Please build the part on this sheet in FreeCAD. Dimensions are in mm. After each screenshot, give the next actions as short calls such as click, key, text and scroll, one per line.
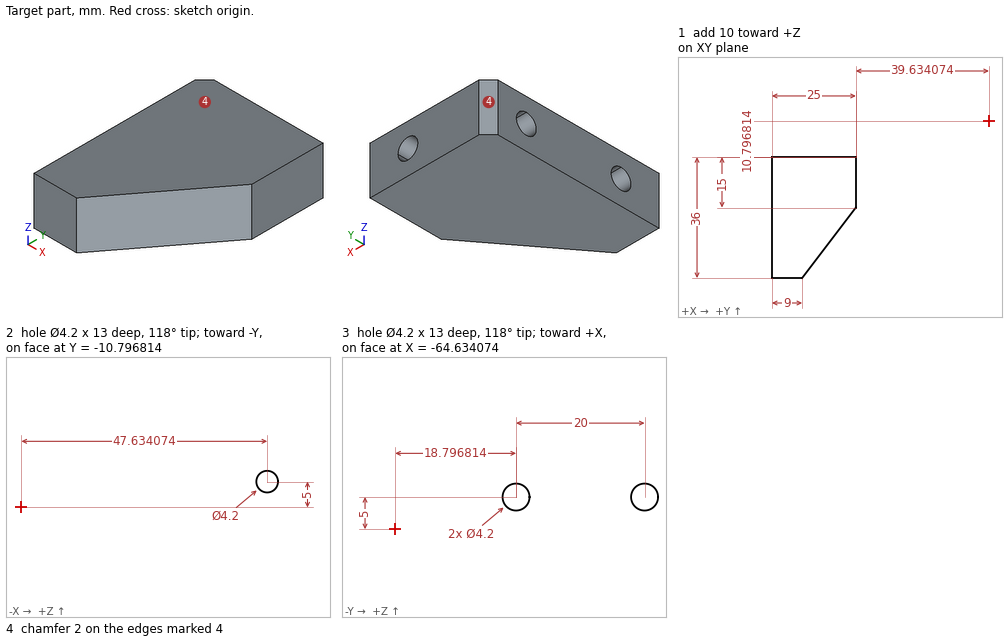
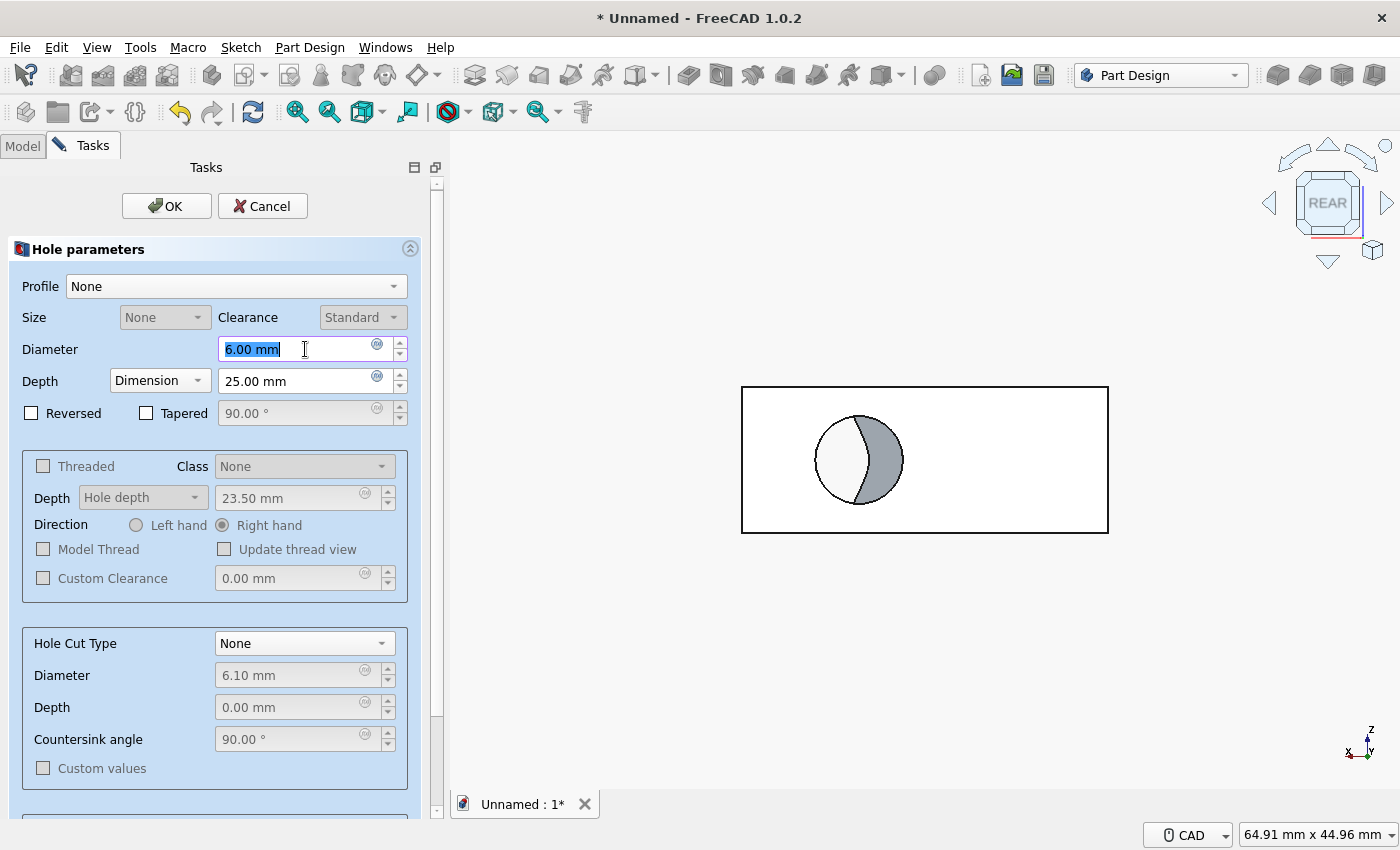
text(4.2)
key(Tab)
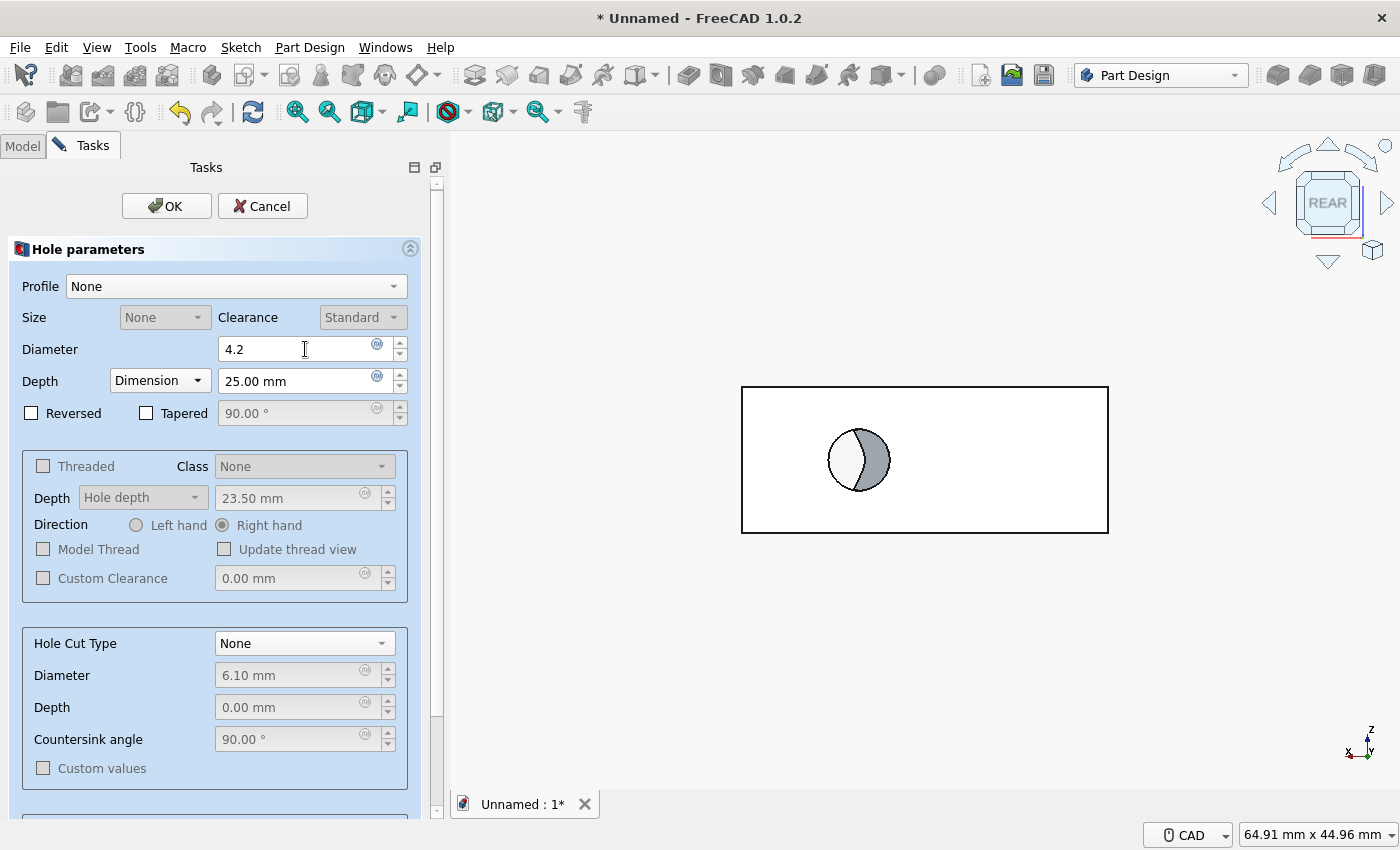
triple_click(305, 381)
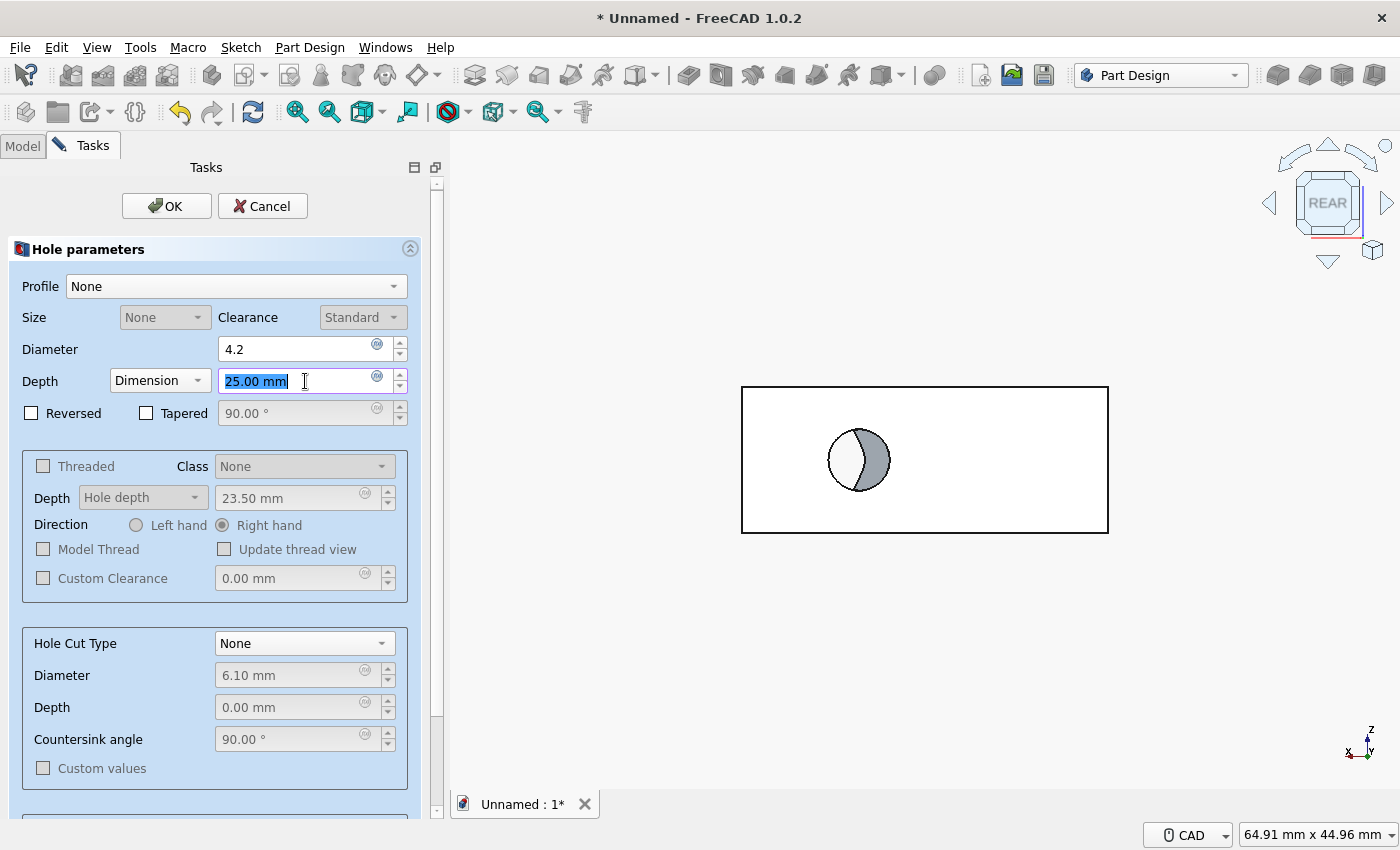
text(13)
key(Tab)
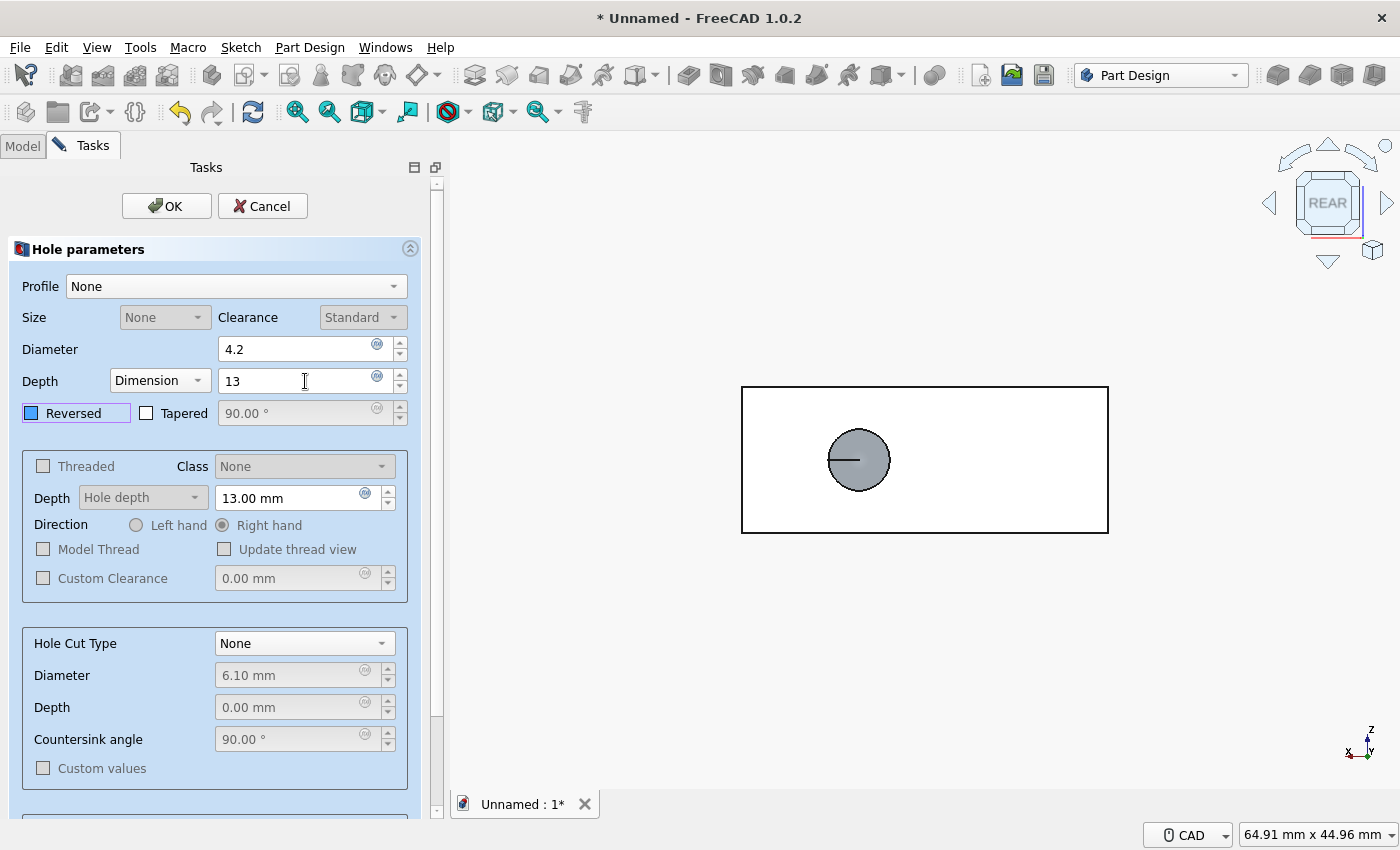
click(167, 206)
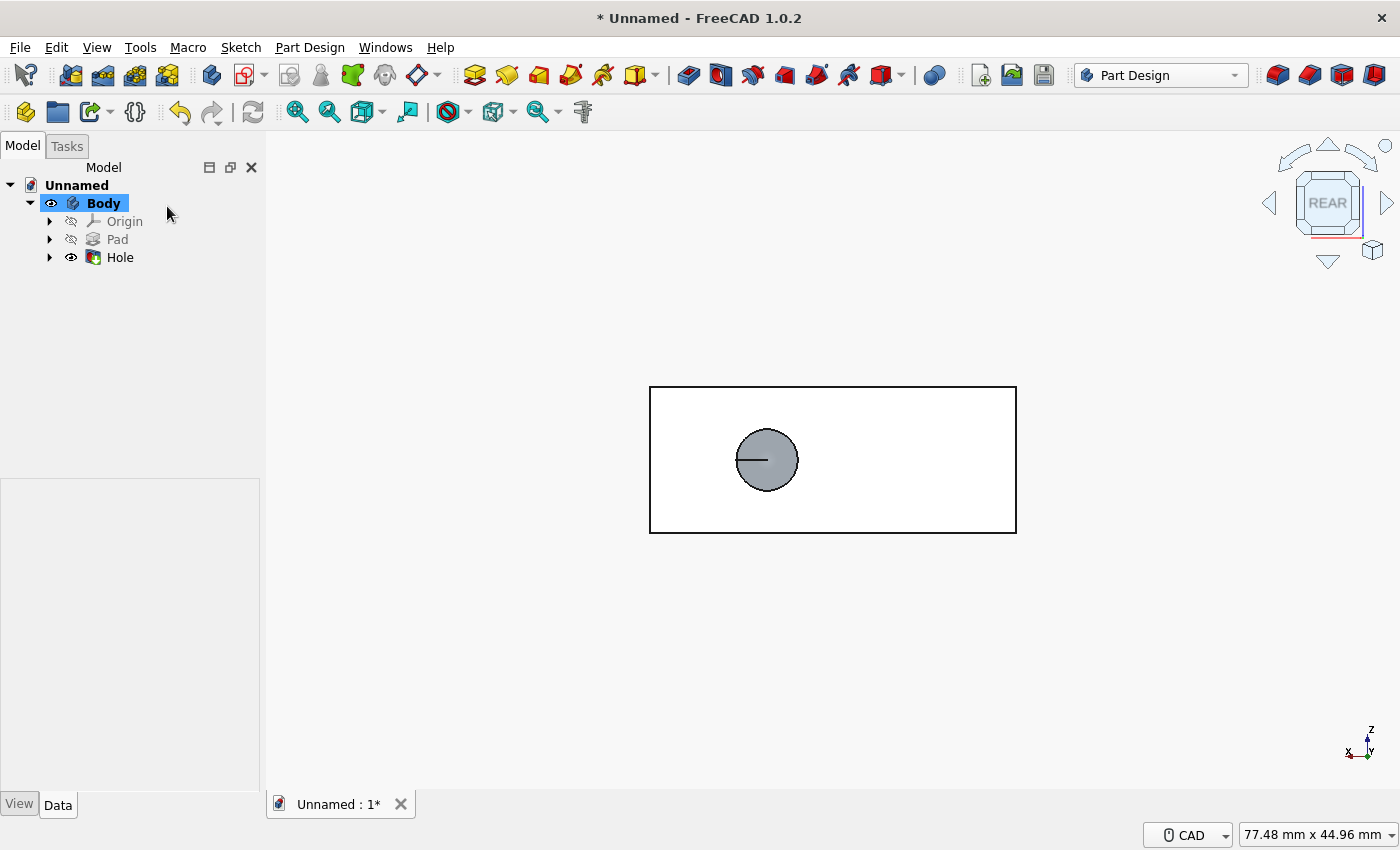
click(298, 112)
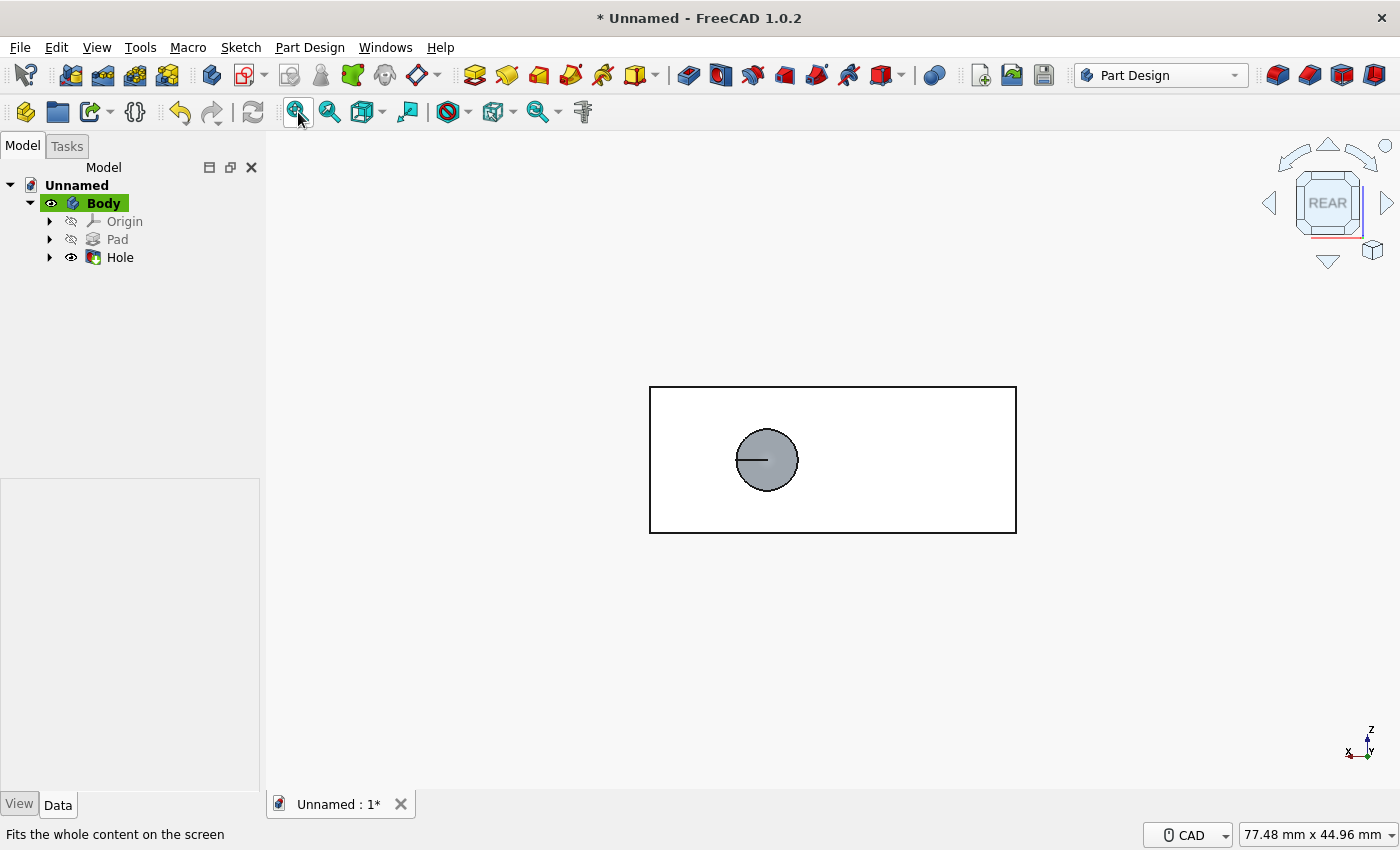
key(6)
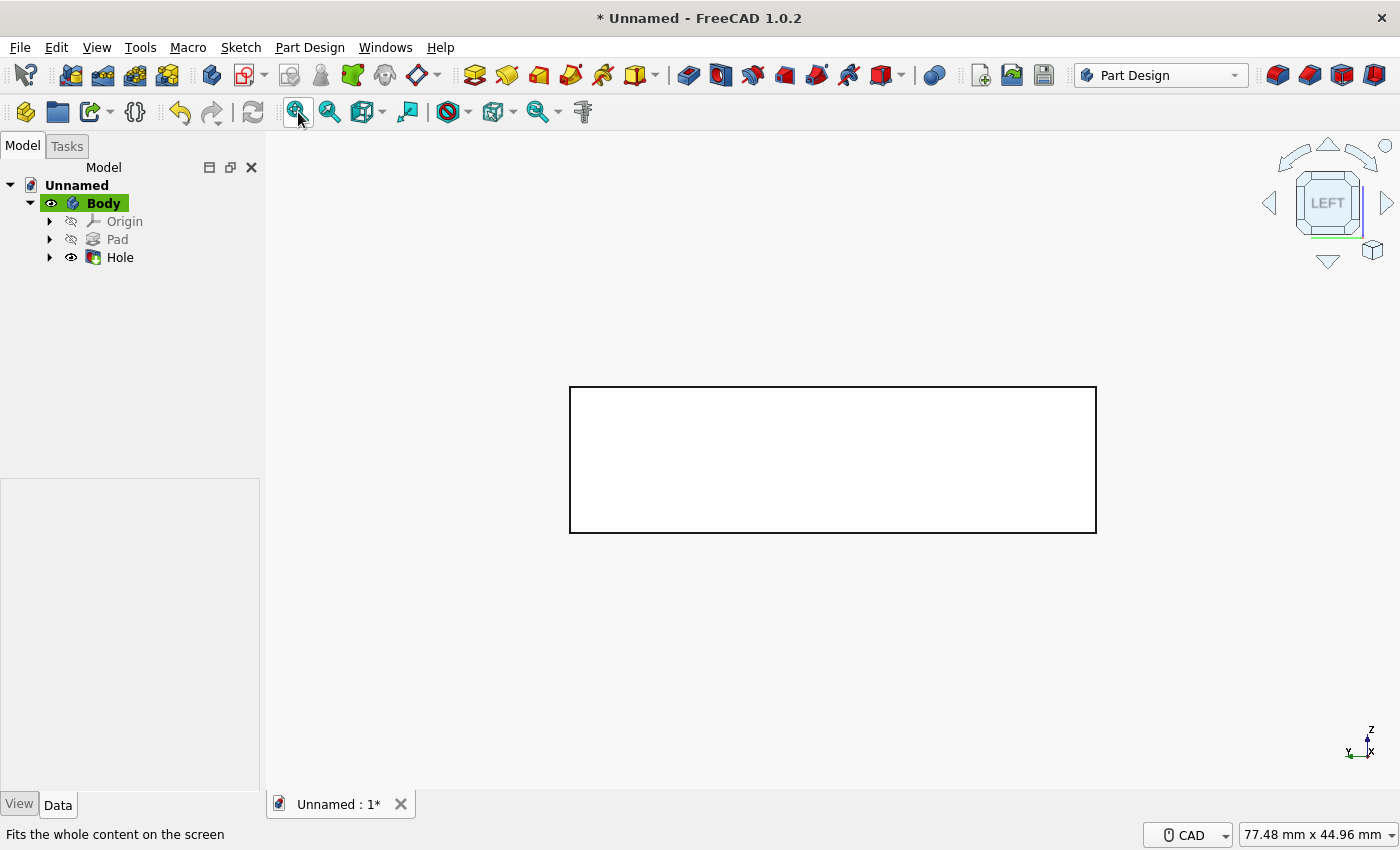
click(682, 459)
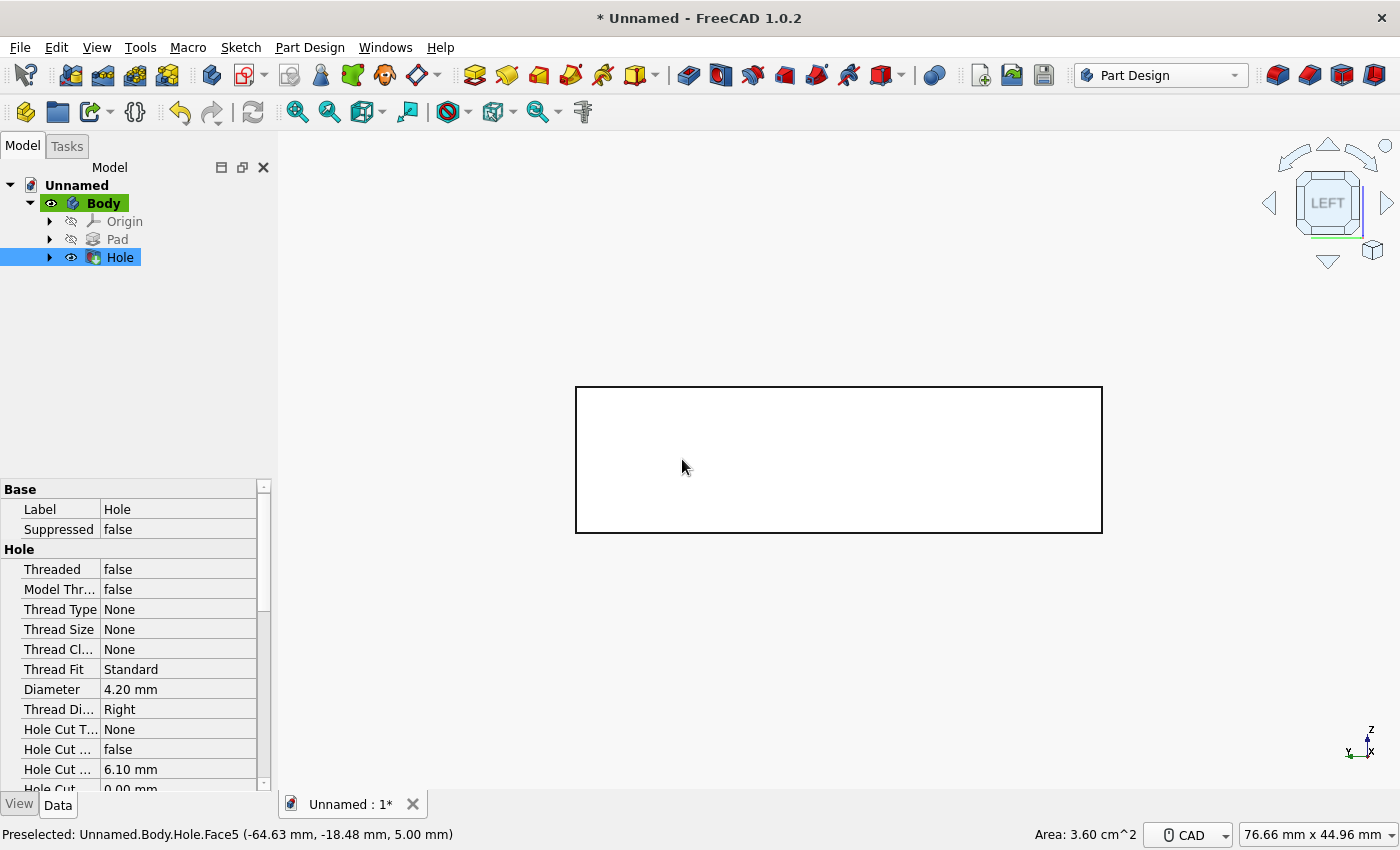
click(244, 76)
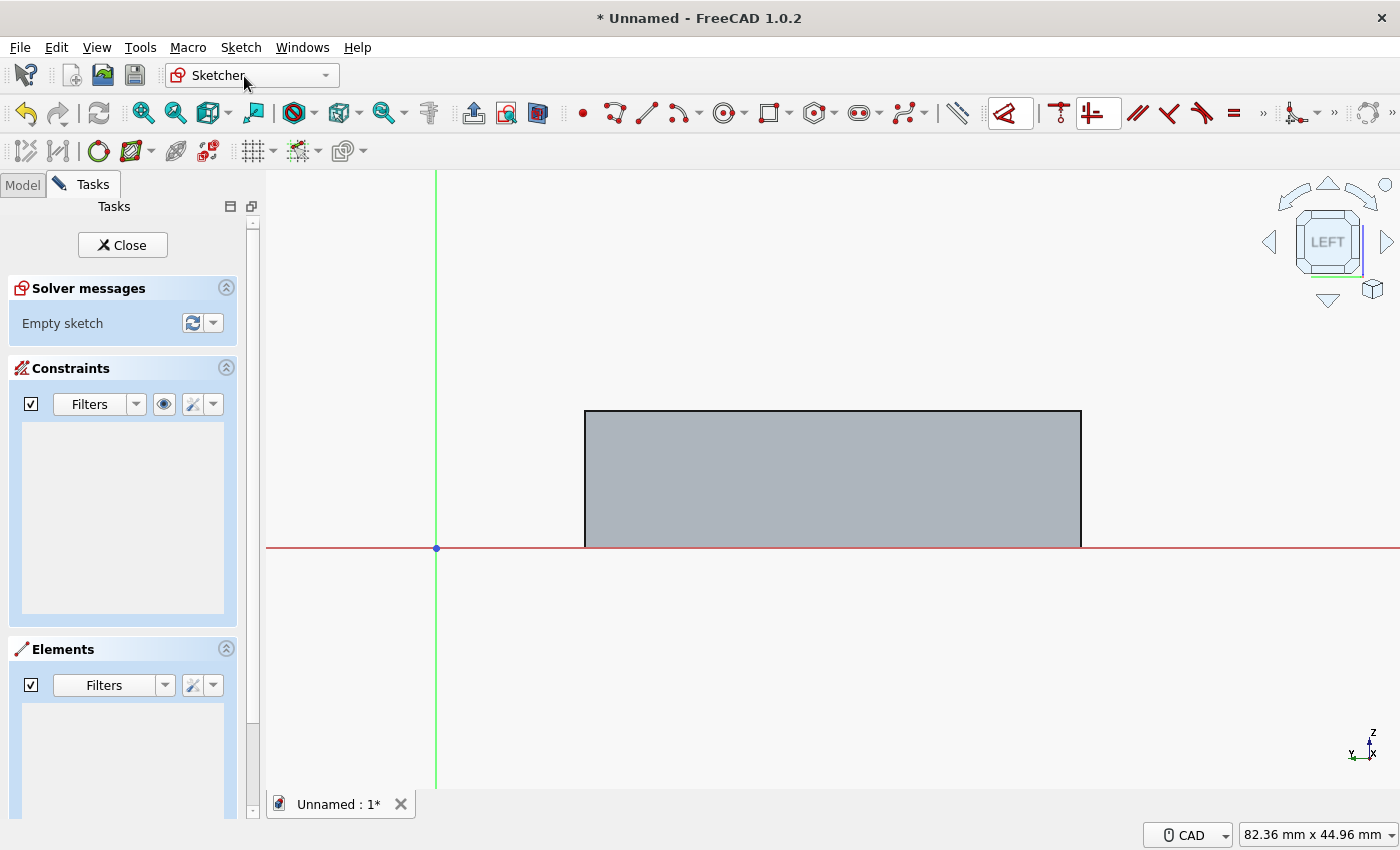
click(724, 114)